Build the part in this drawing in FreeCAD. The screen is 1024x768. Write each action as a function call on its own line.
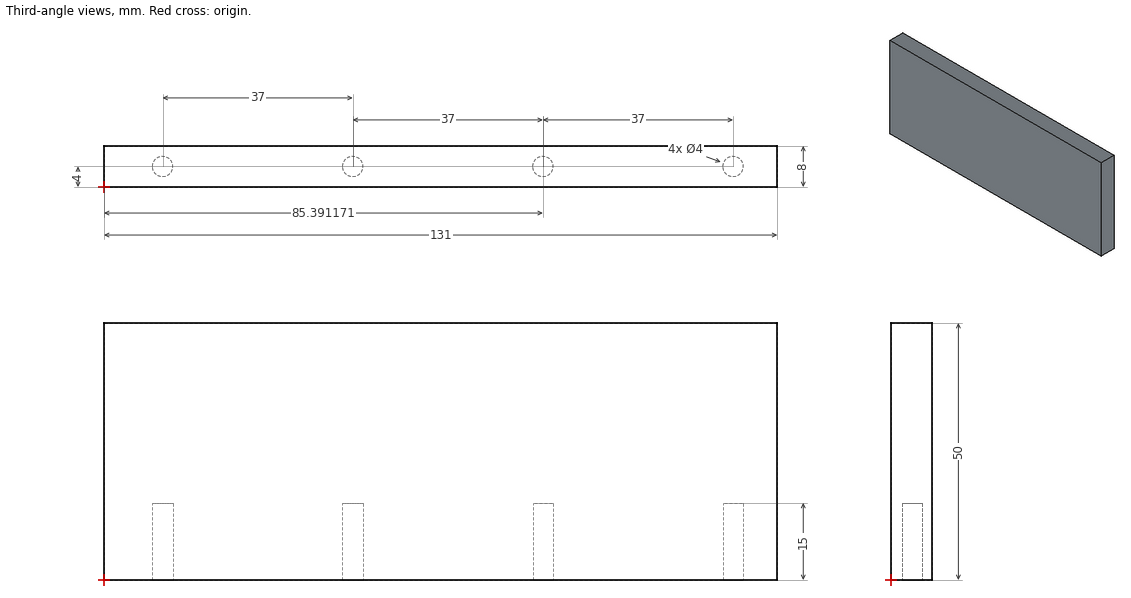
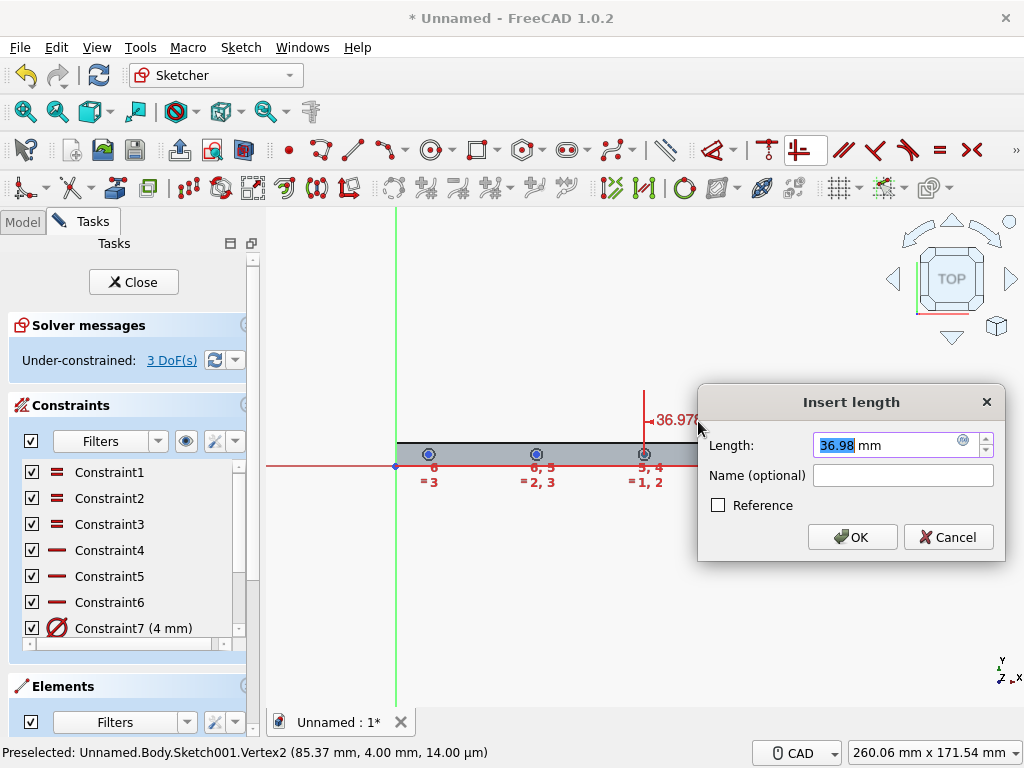
text(37)
key(Return)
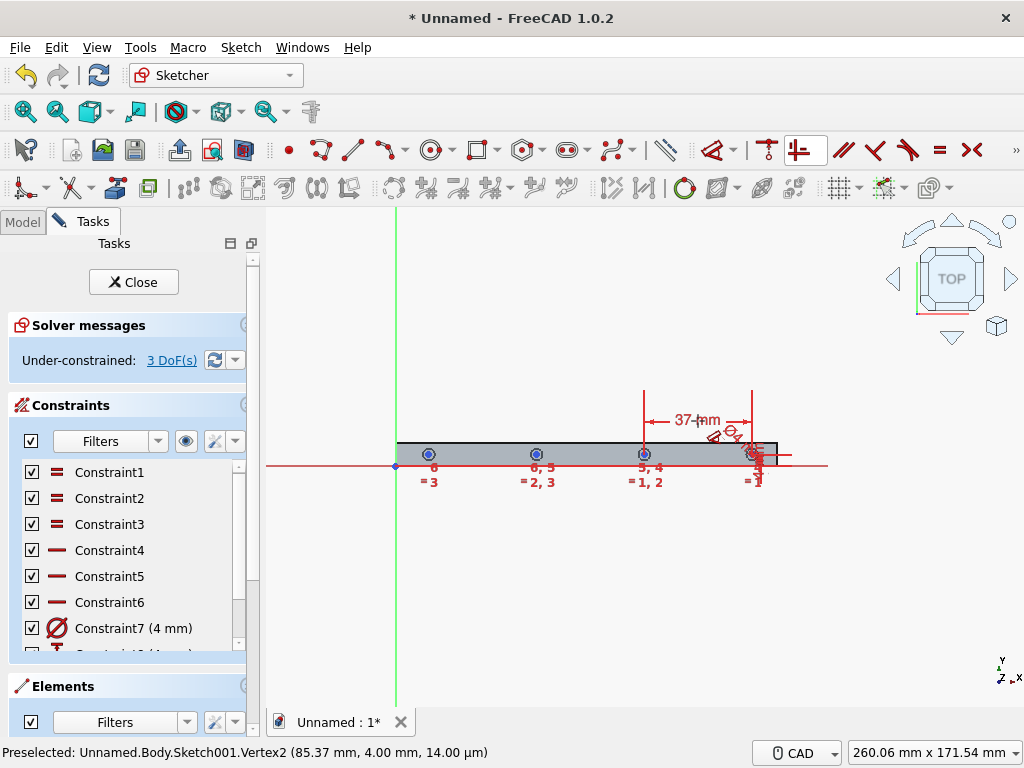
click(644, 455)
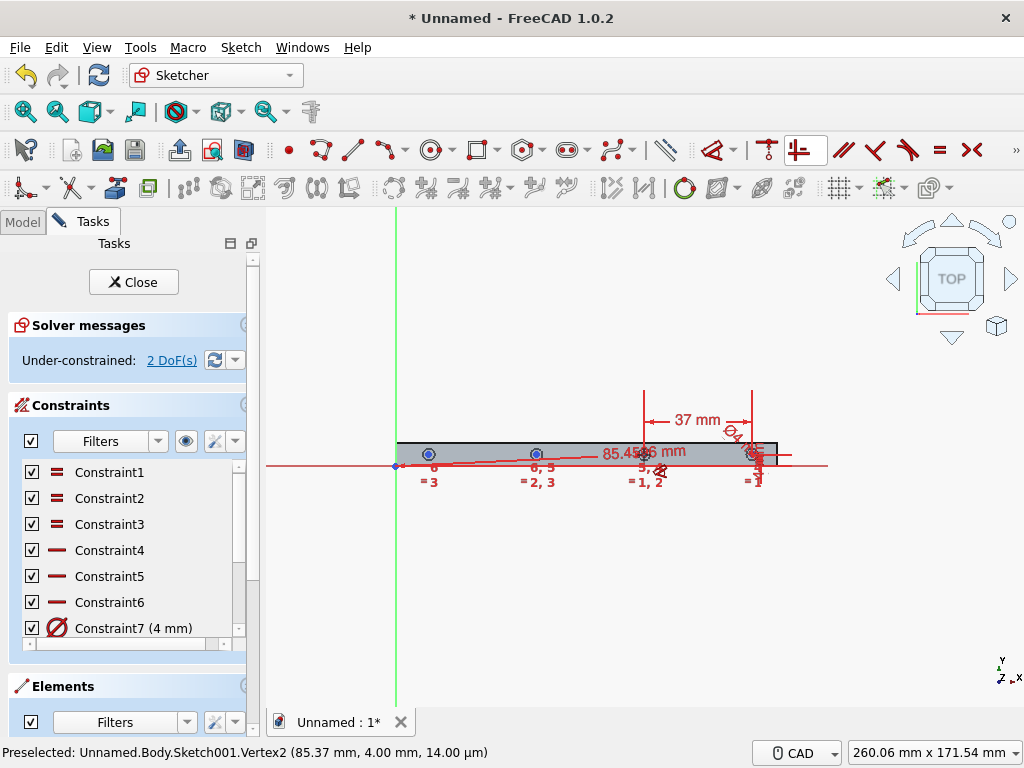
click(537, 455)
click(591, 421)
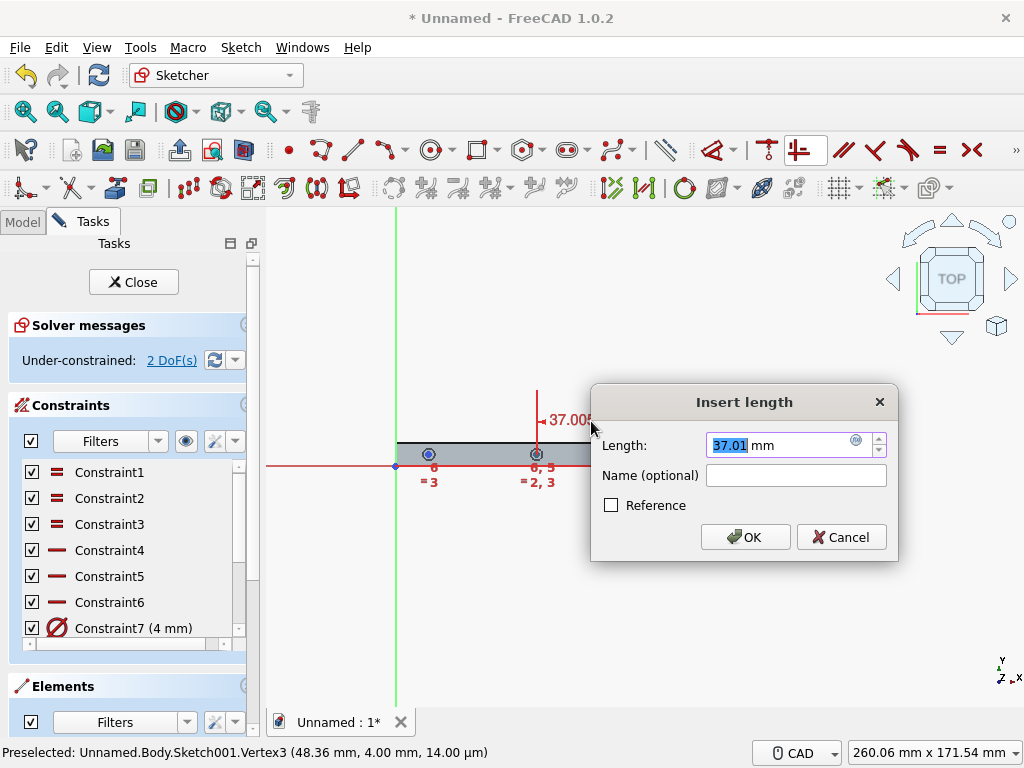
text(37)
key(Return)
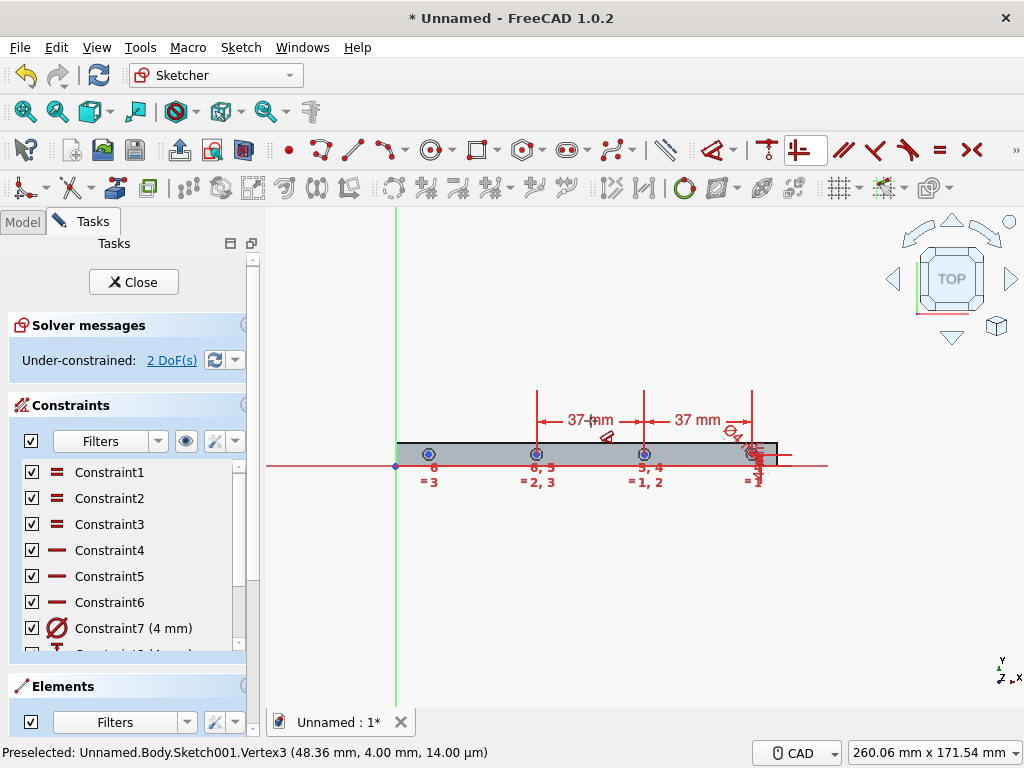
click(537, 455)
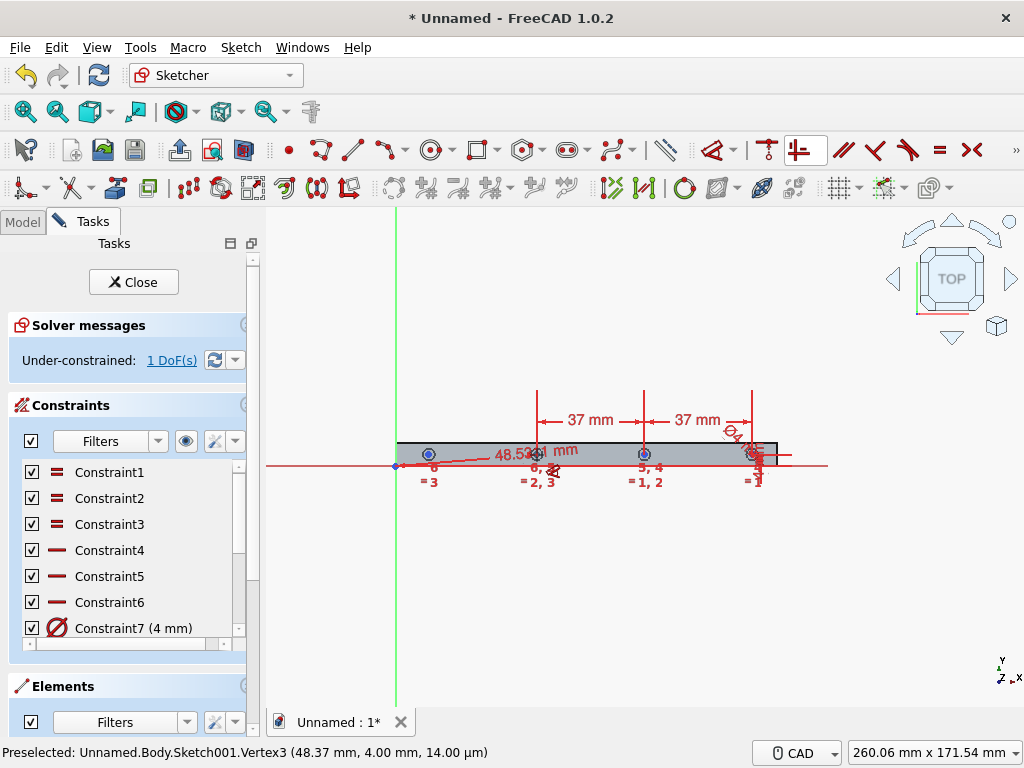
click(429, 455)
click(483, 421)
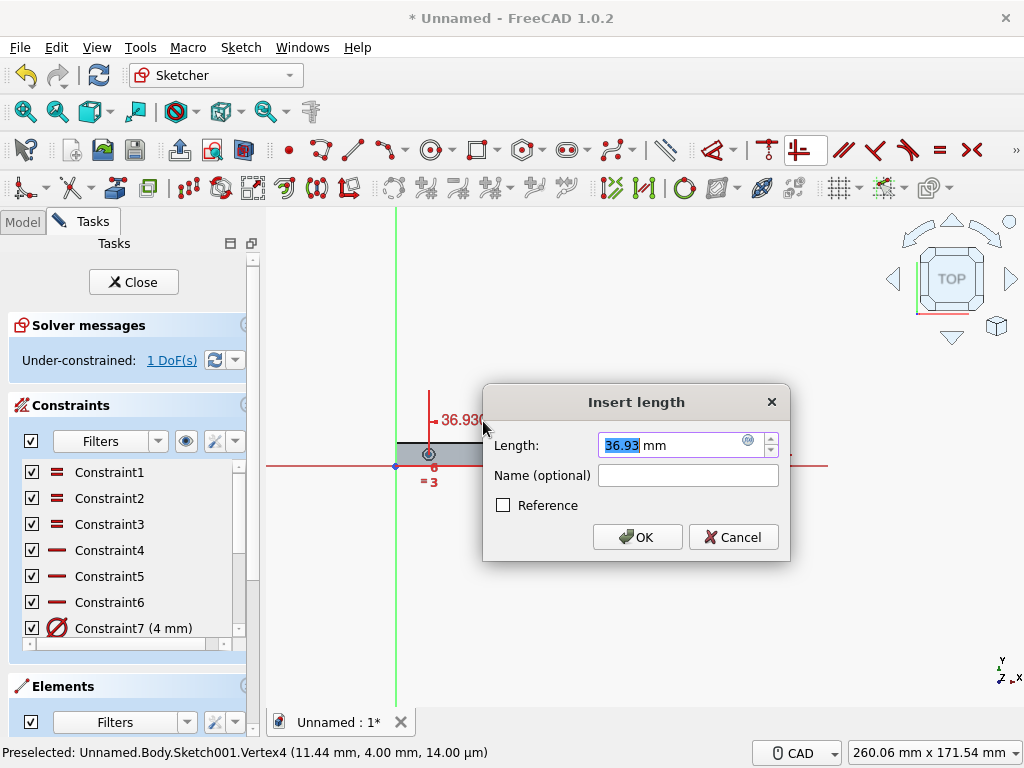
text(37)
key(Return)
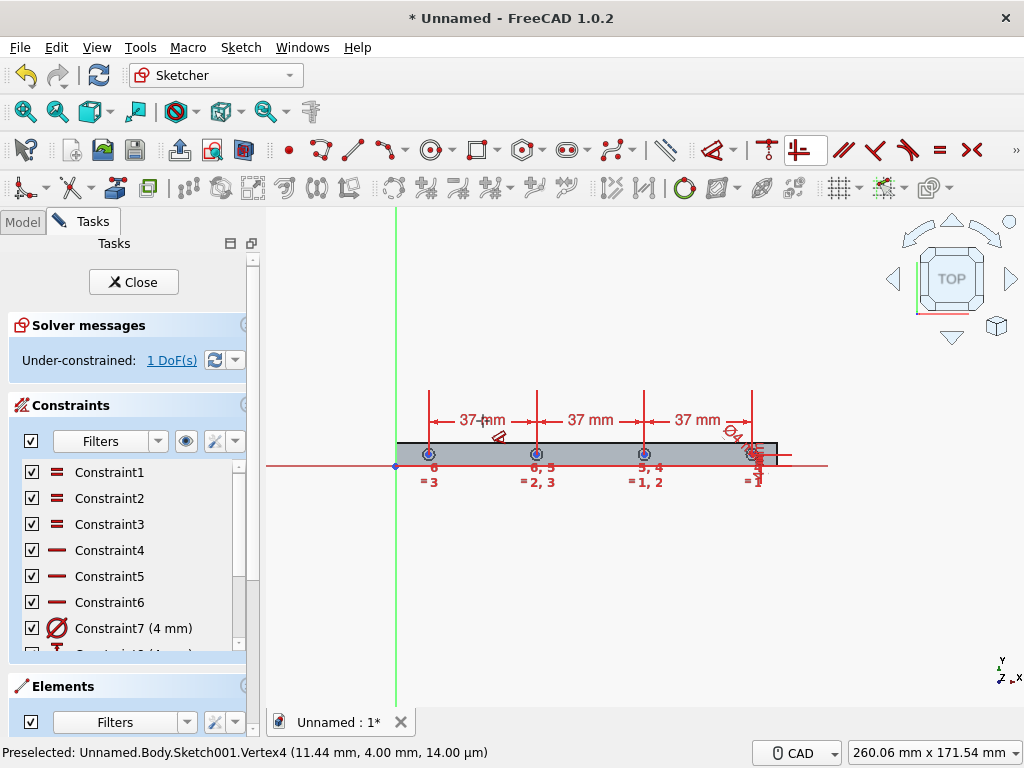
click(644, 455)
click(520, 500)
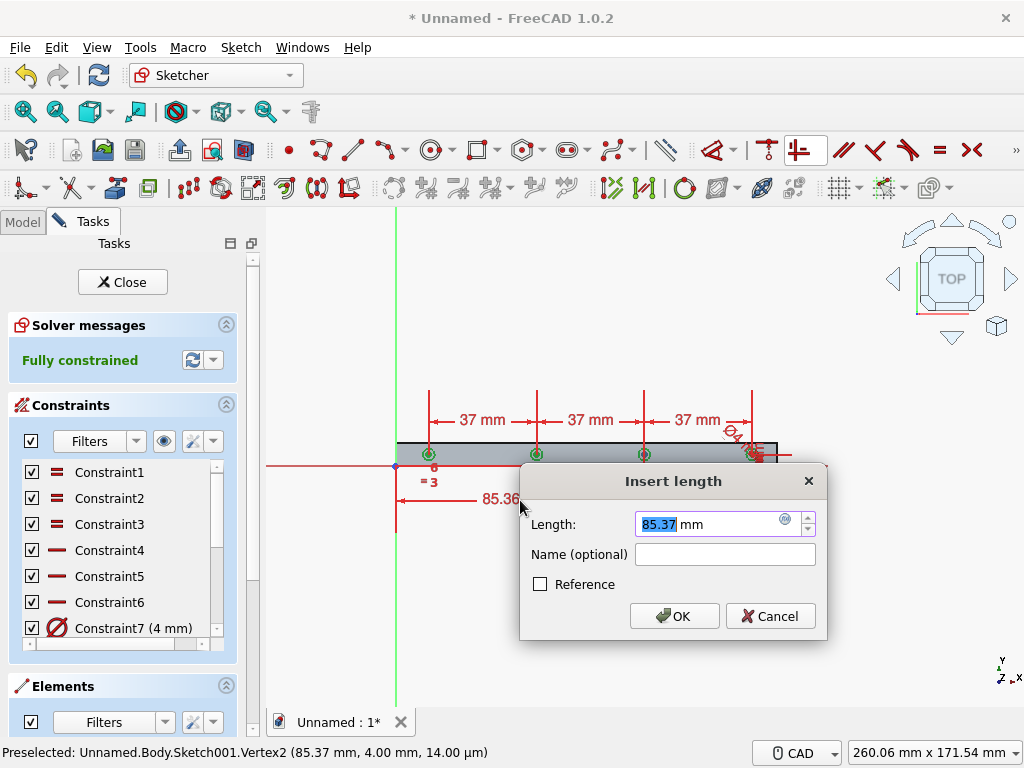
text(85.391171)
key(Return)
key(Escape)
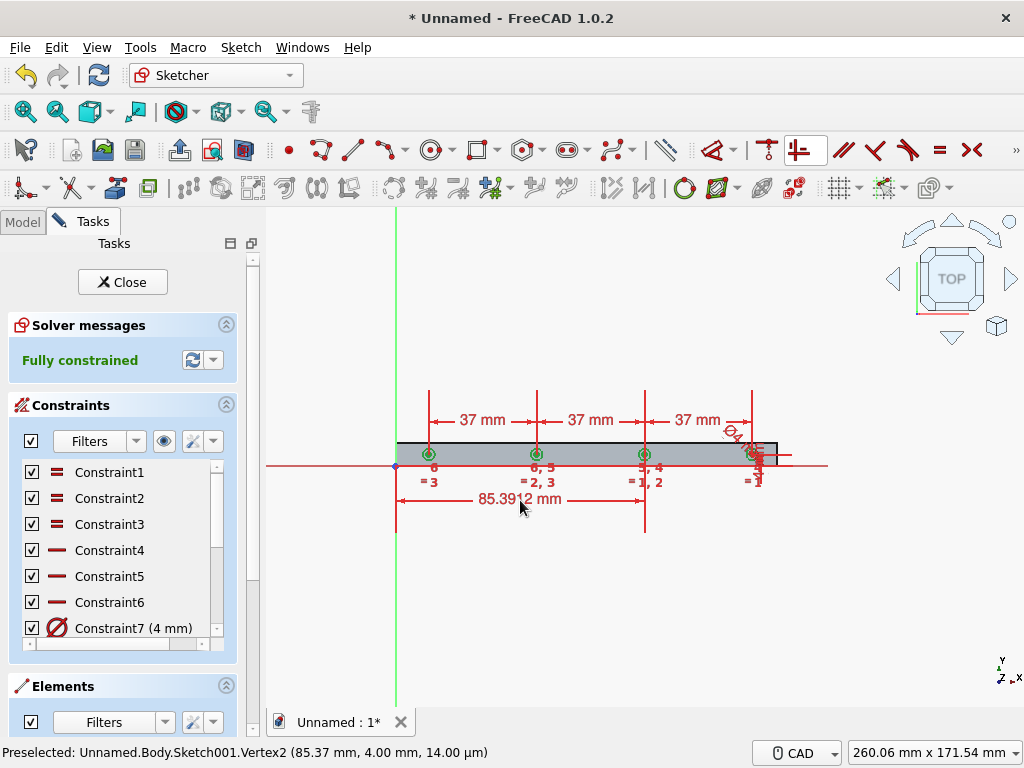
click(123, 282)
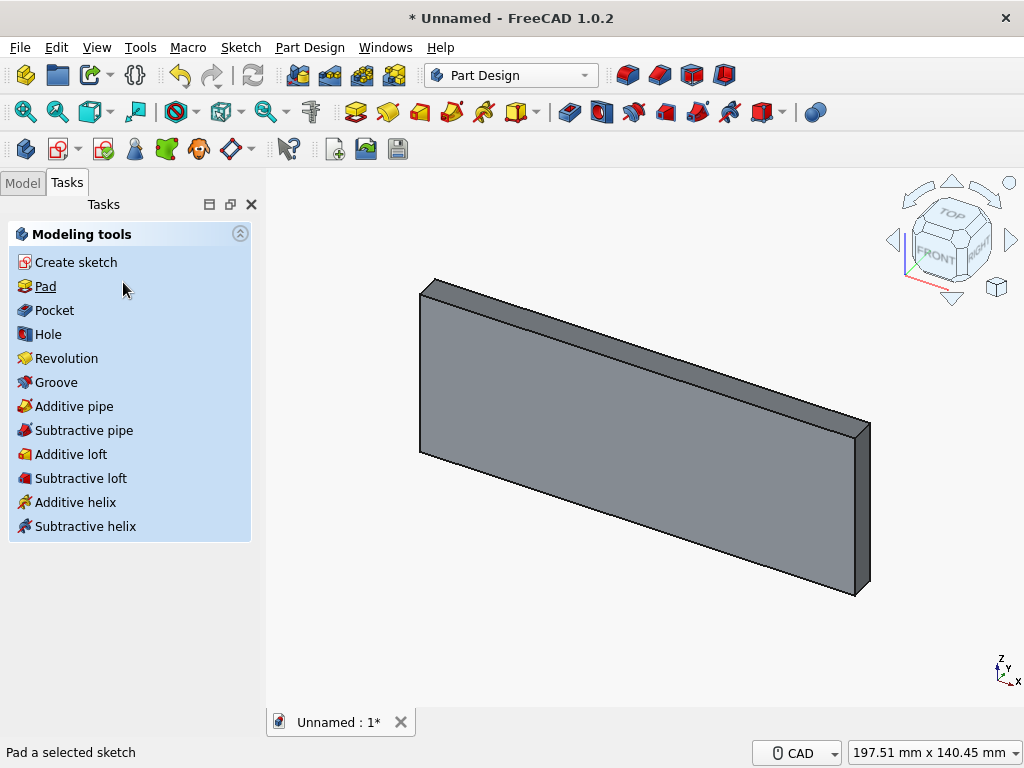
click(570, 112)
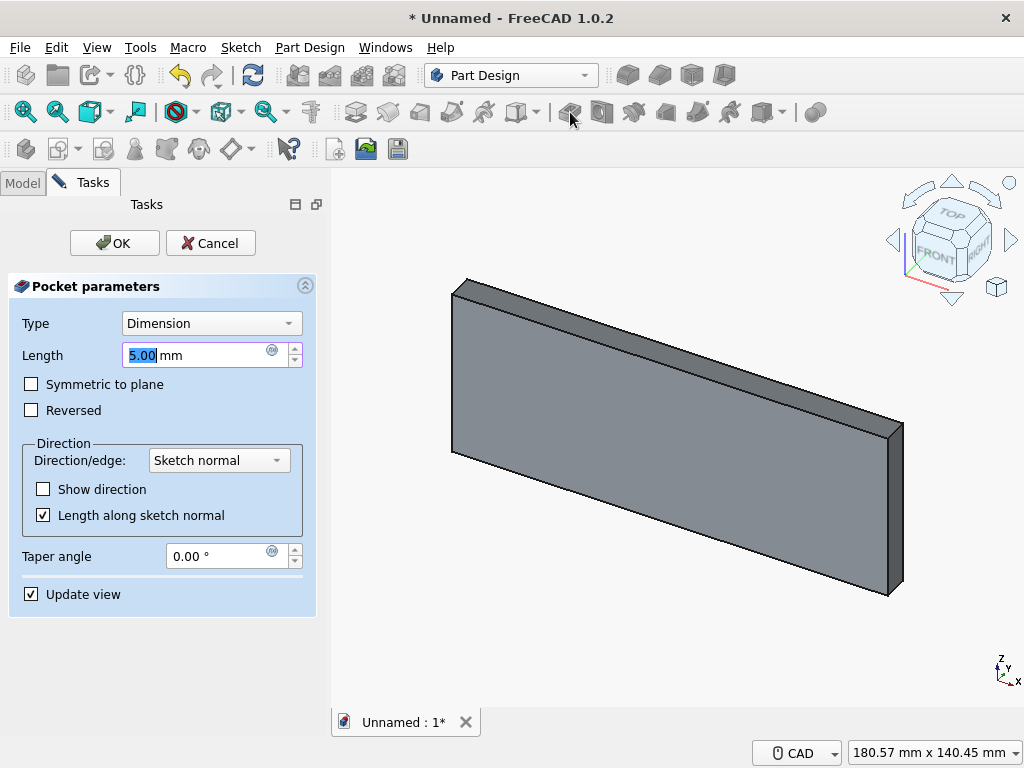
text(15)
key(Tab)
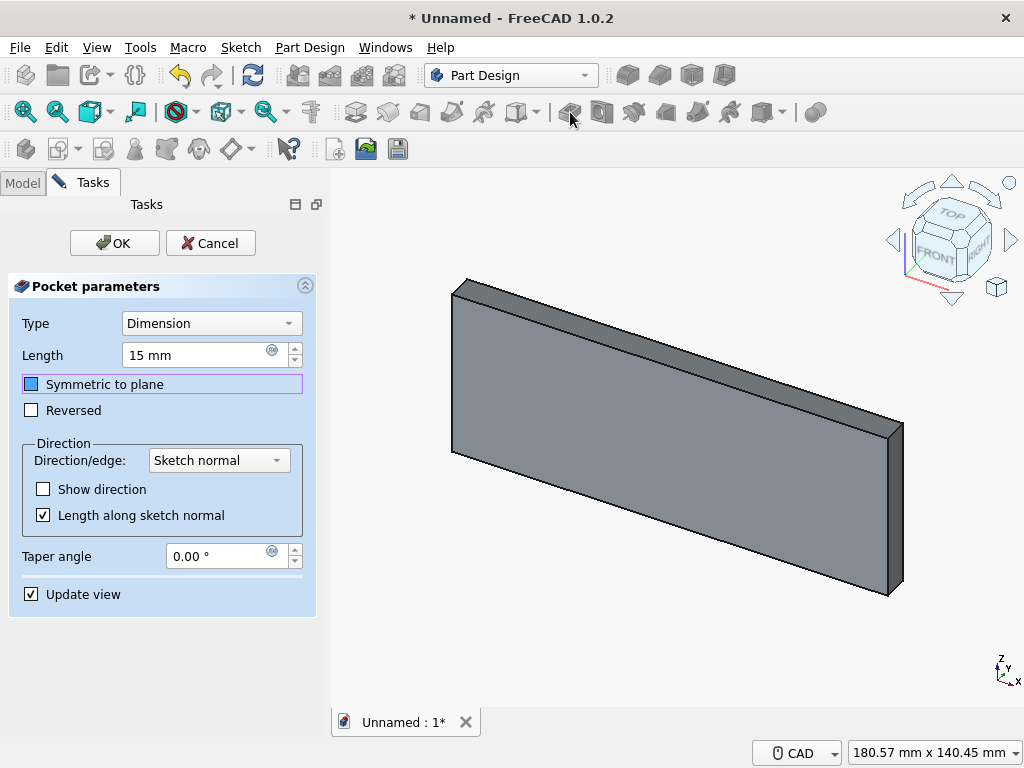
click(30, 410)